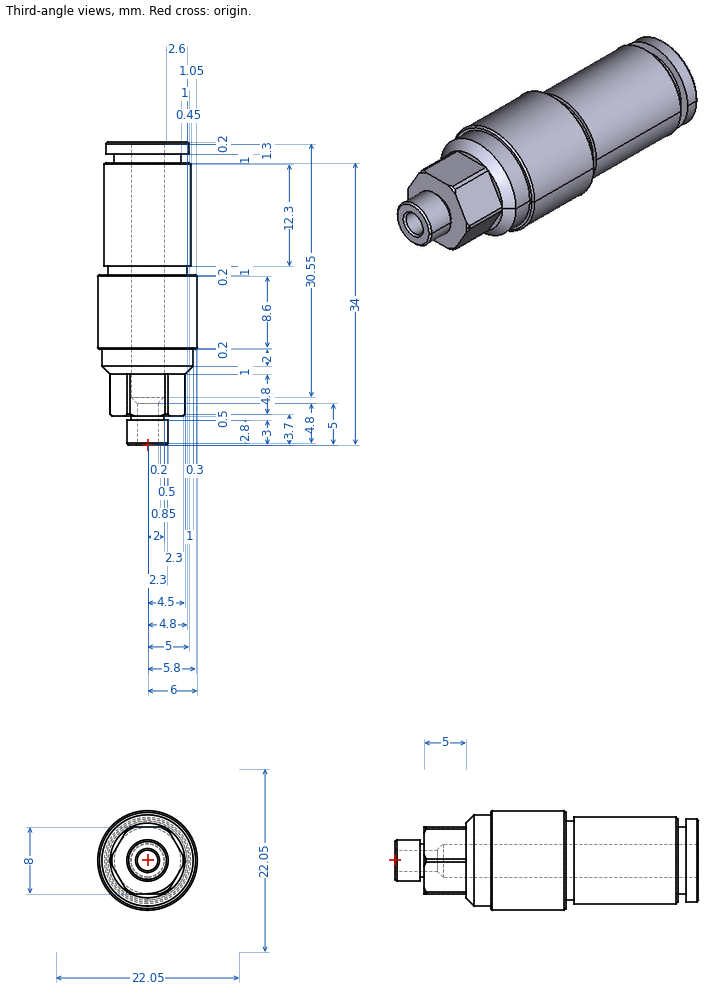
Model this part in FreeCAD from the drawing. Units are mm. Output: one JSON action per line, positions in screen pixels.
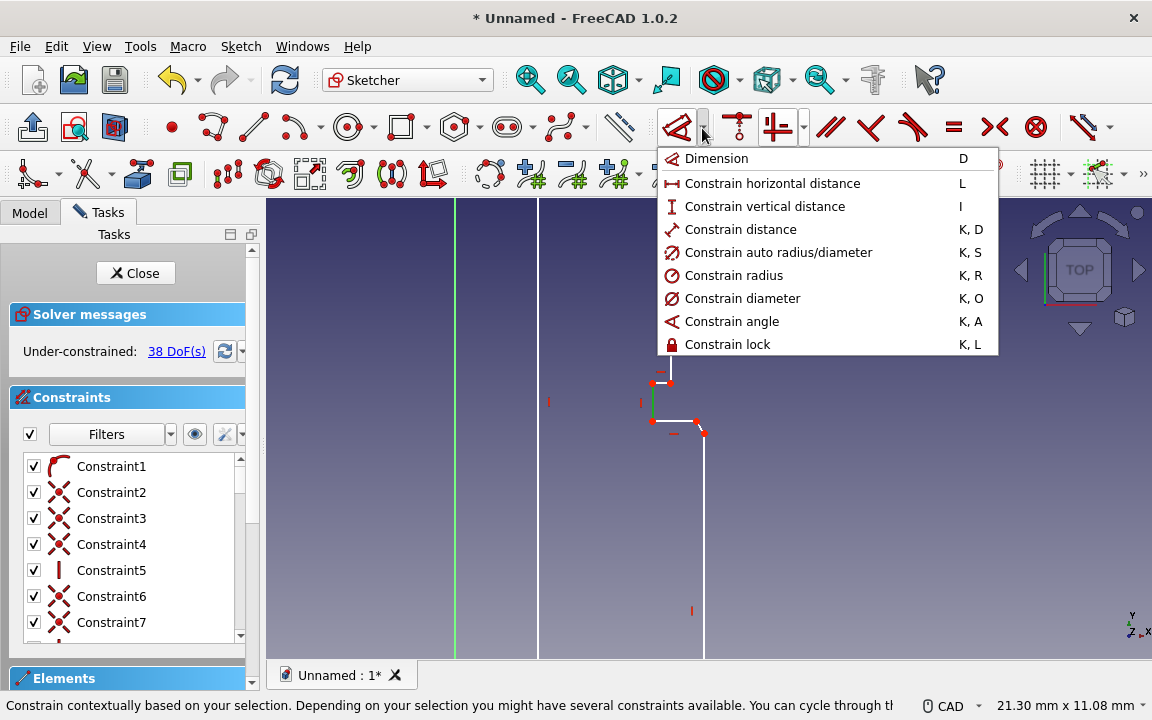
{"action": "left_click", "coordinate": [828, 206]}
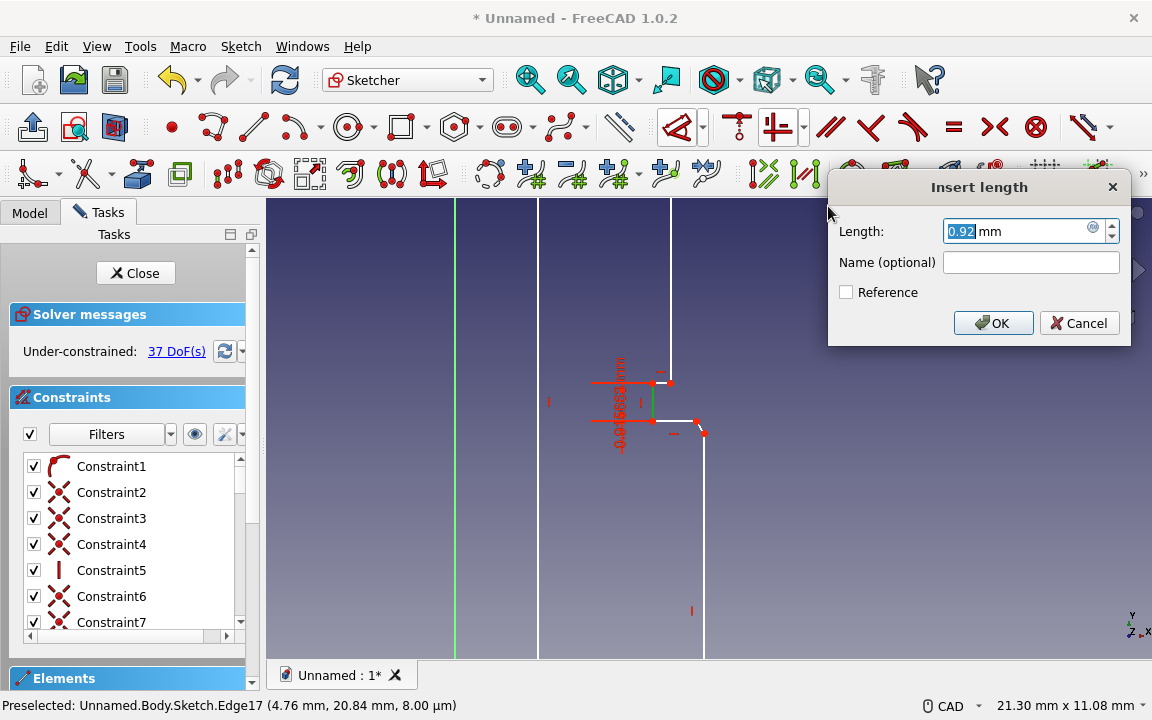
{"action": "type", "text": "1"}
{"action": "key", "text": "Return"}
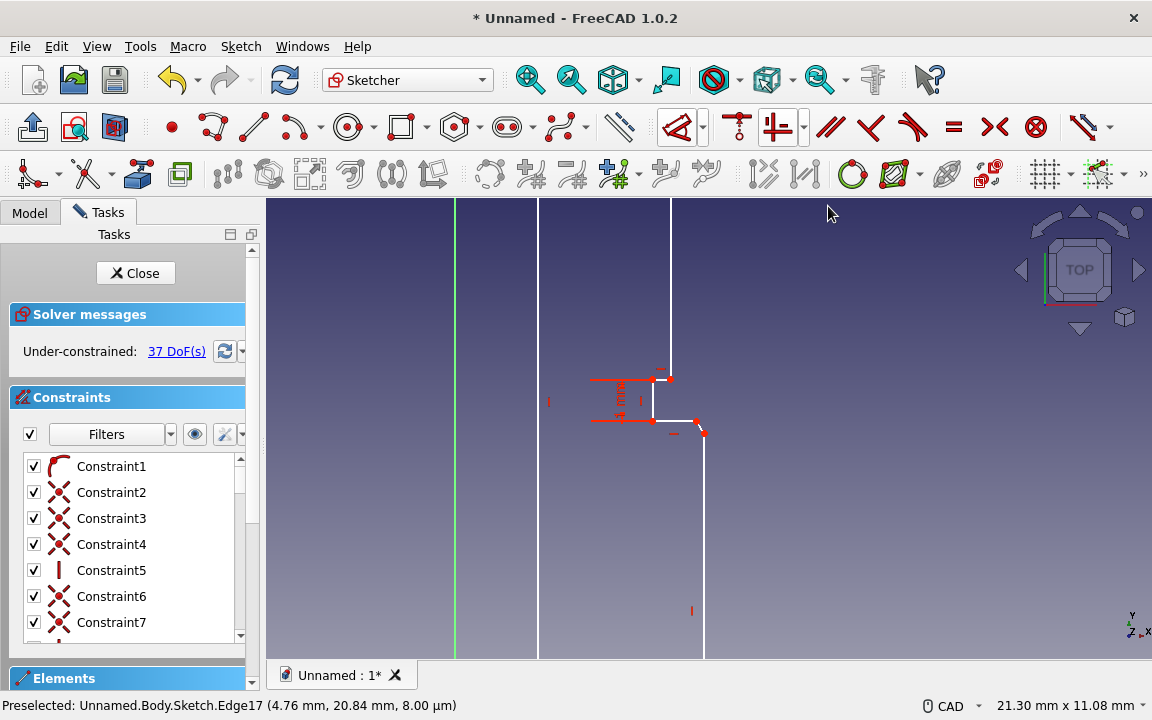
{"action": "scroll", "coordinate": [656, 407], "scroll_direction": "down", "scroll_amount": 8}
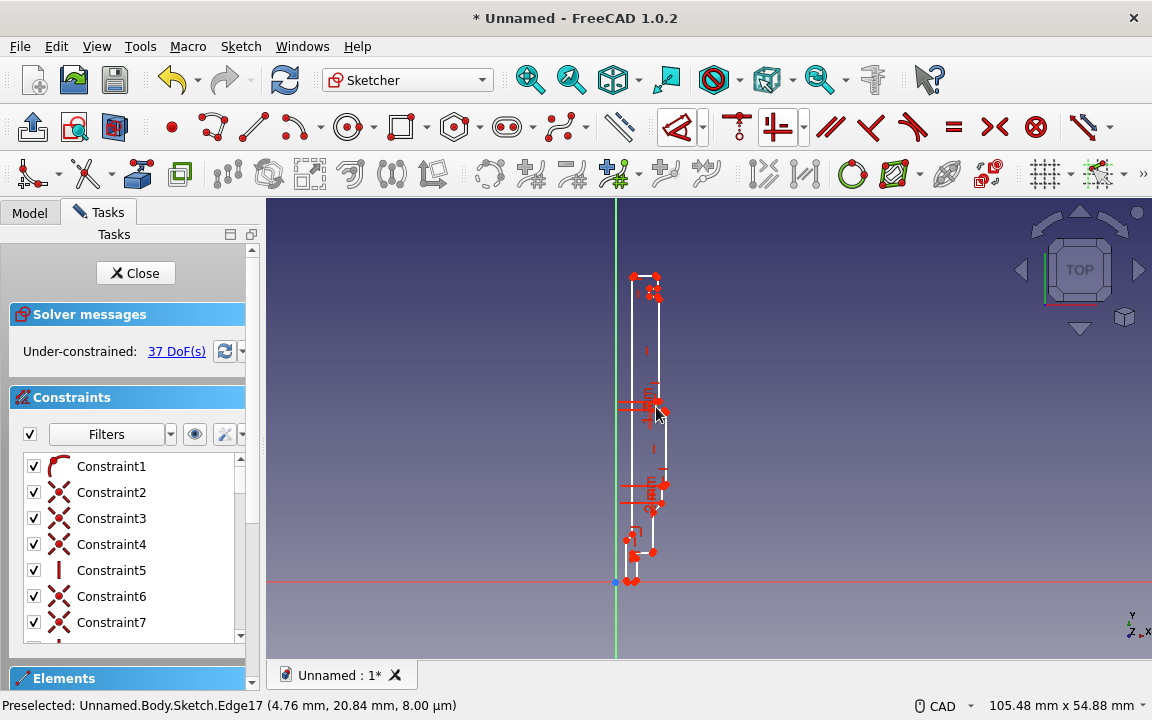
{"action": "scroll", "coordinate": [655, 297], "scroll_direction": "up", "scroll_amount": 9}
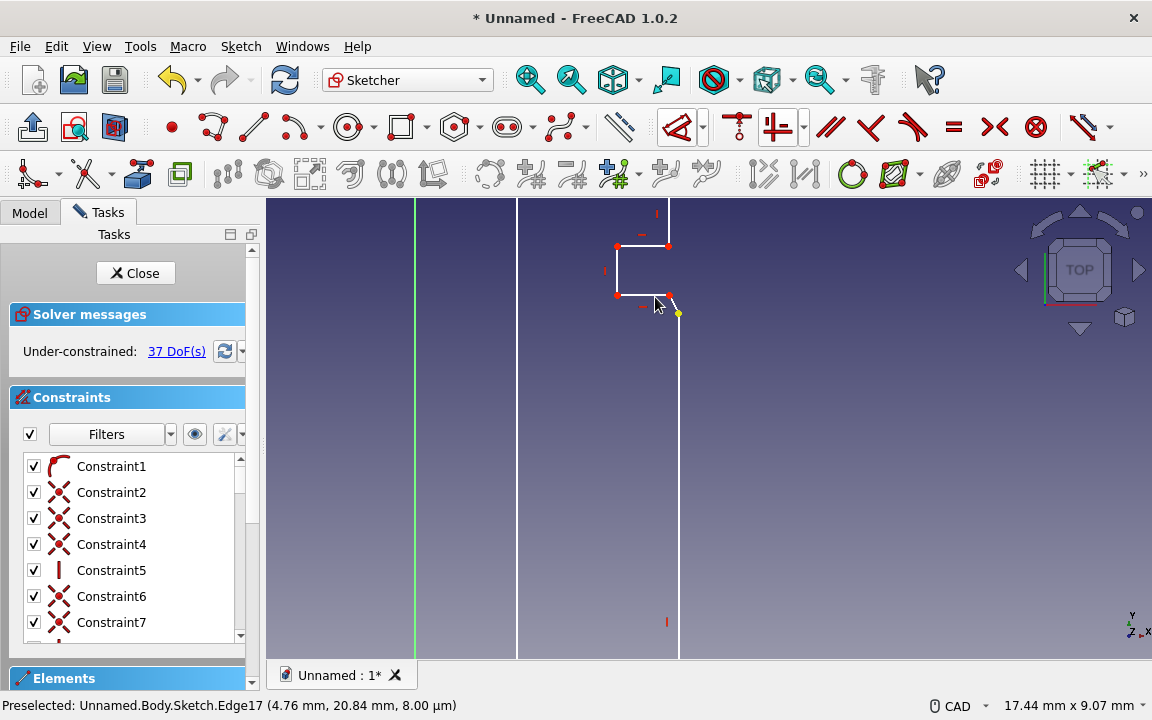
{"action": "left_click", "coordinate": [654, 295]}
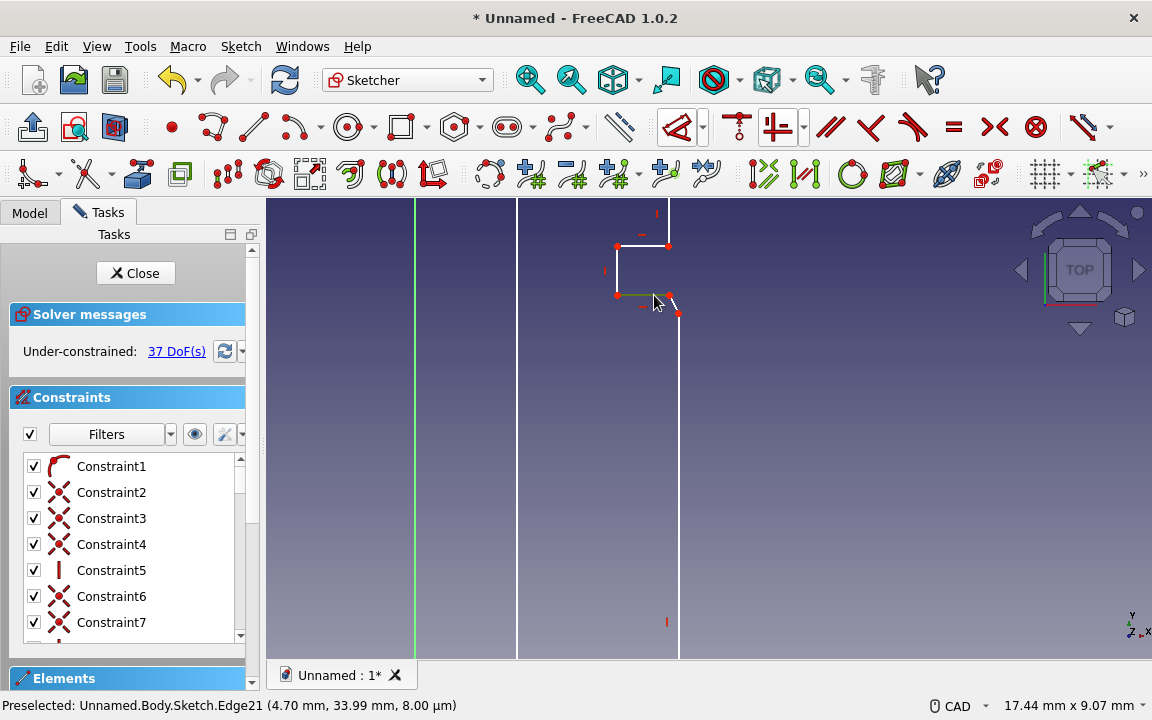
{"action": "key", "text": "l"}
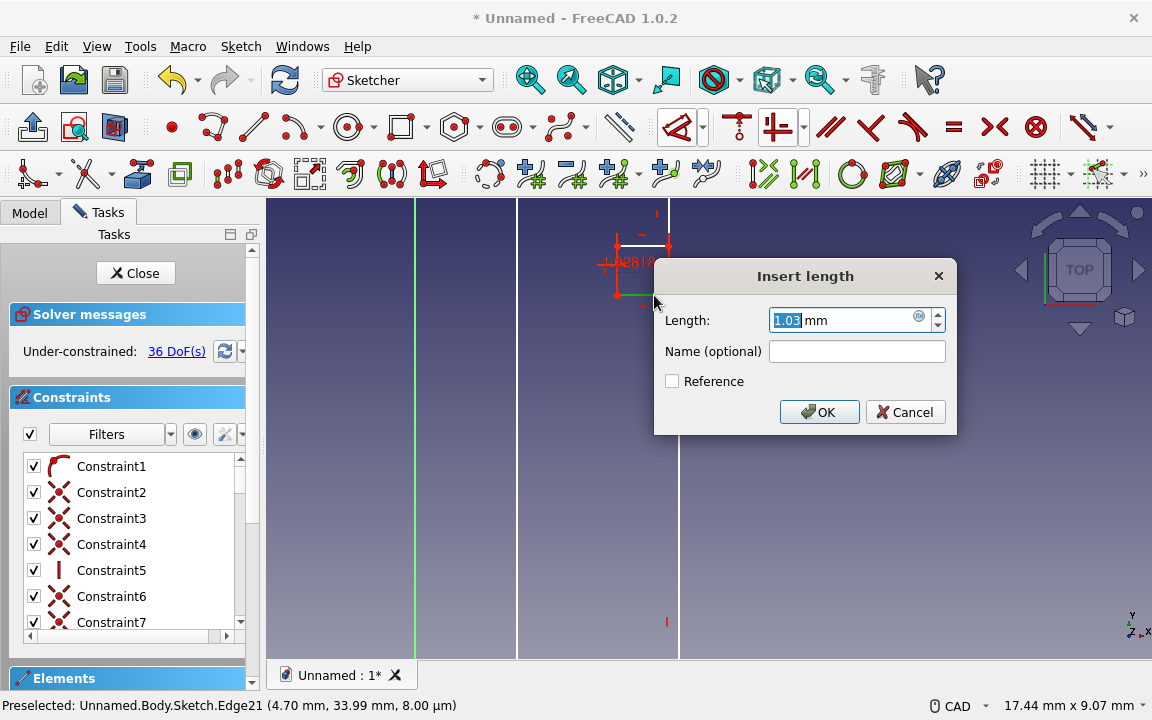
{"action": "type", "text": "1"}
{"action": "key", "text": "Return"}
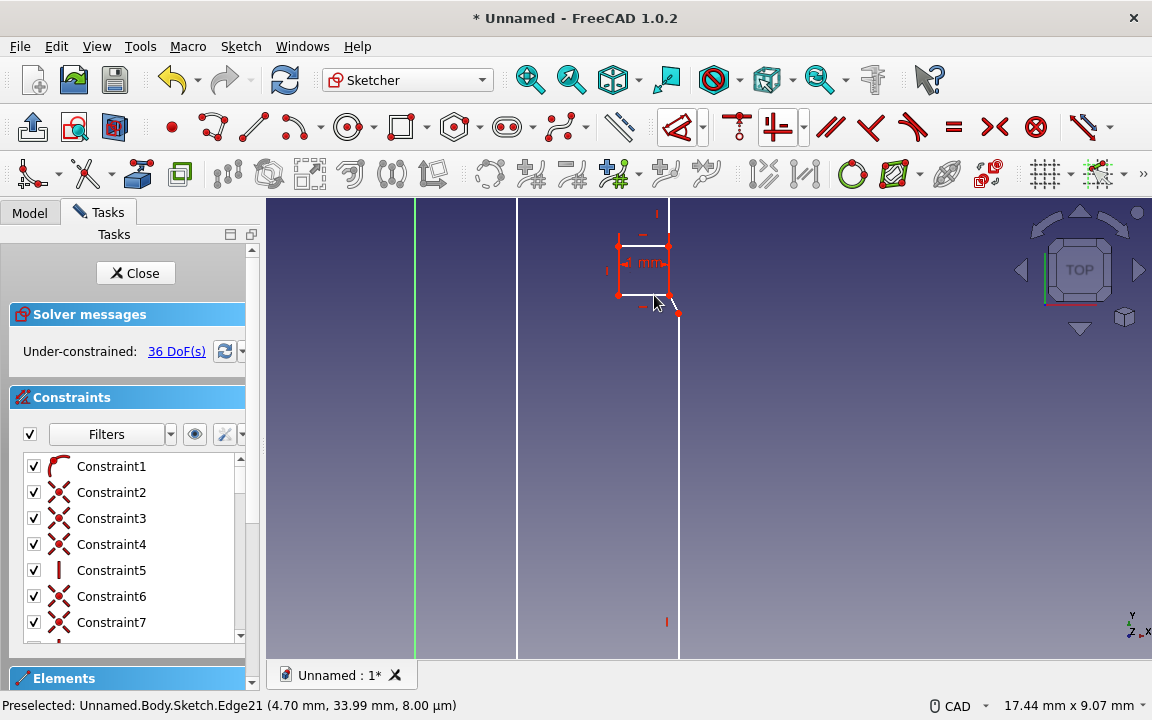
{"action": "left_click", "coordinate": [619, 281]}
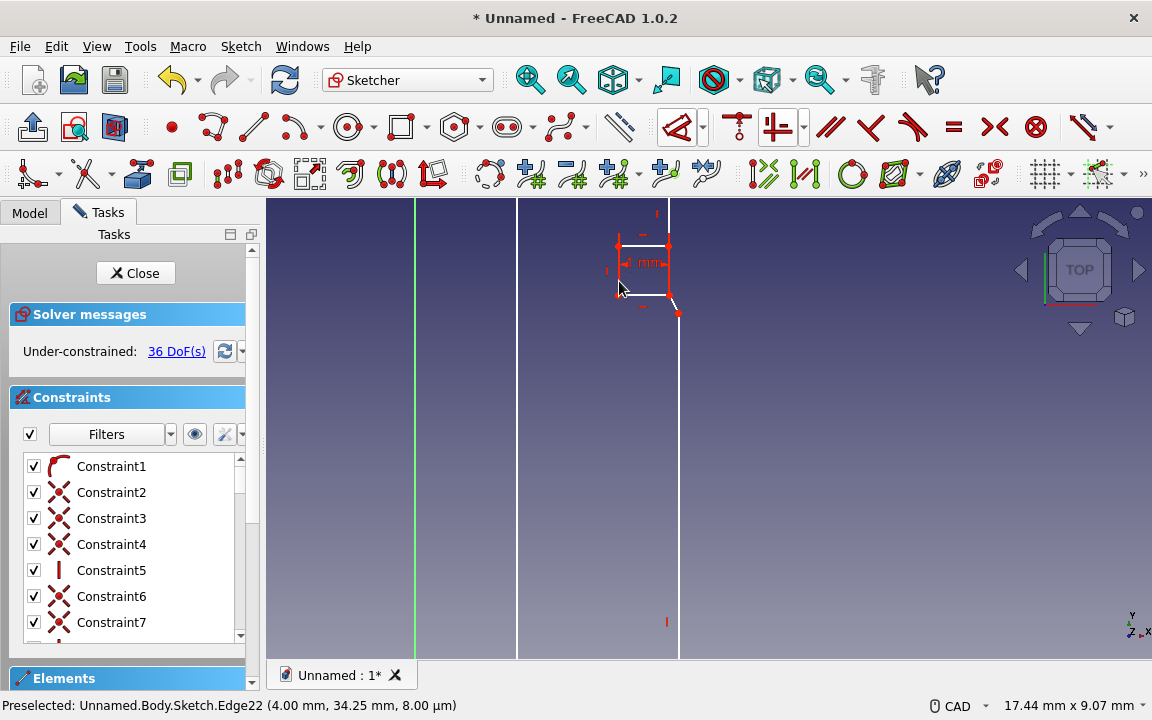
{"action": "left_click", "coordinate": [702, 128]}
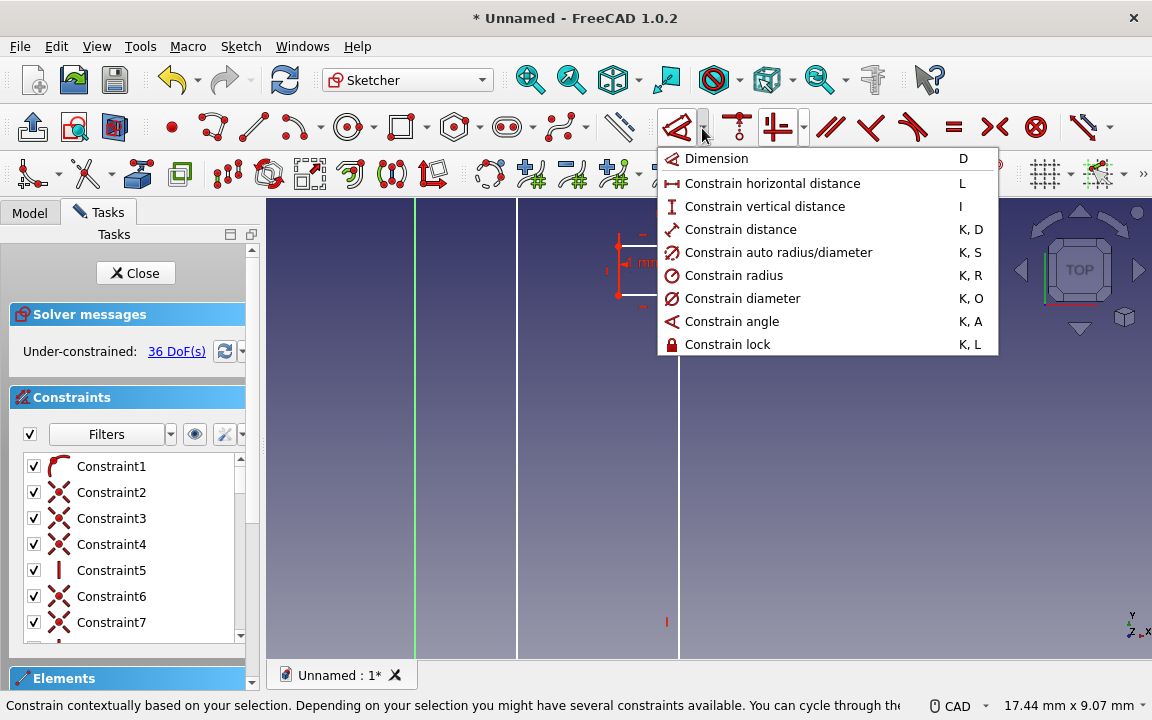
{"action": "left_click", "coordinate": [828, 206]}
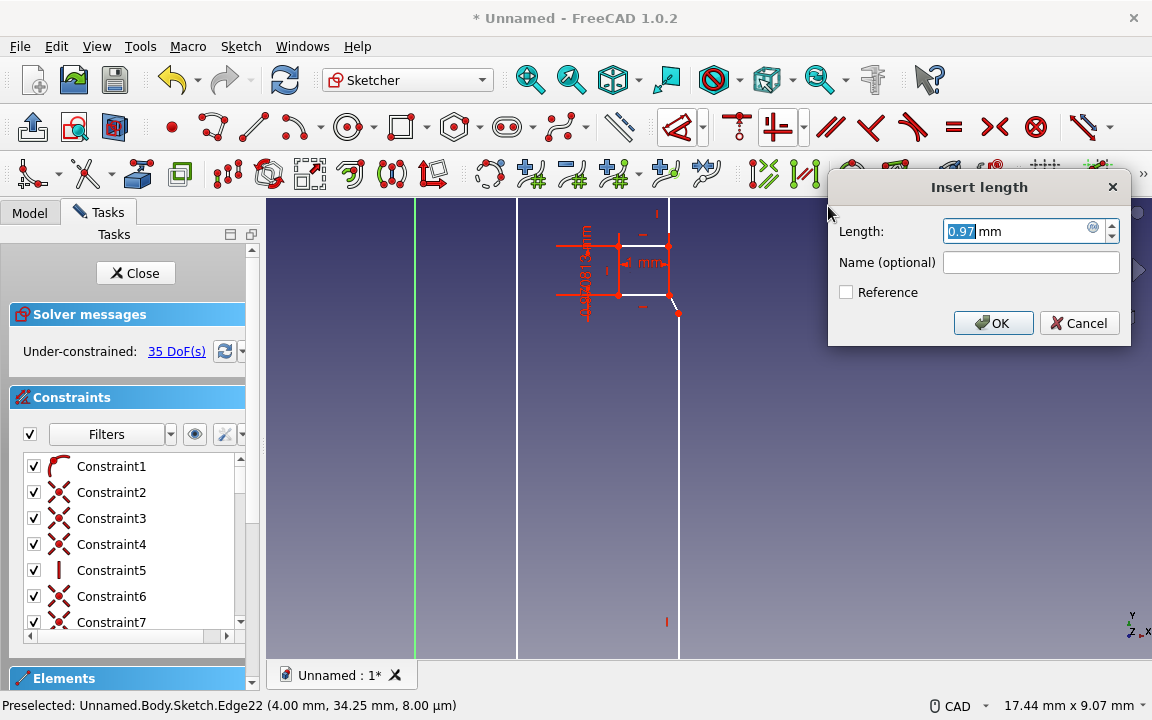
{"action": "type", "text": "1"}
{"action": "key", "text": "Return"}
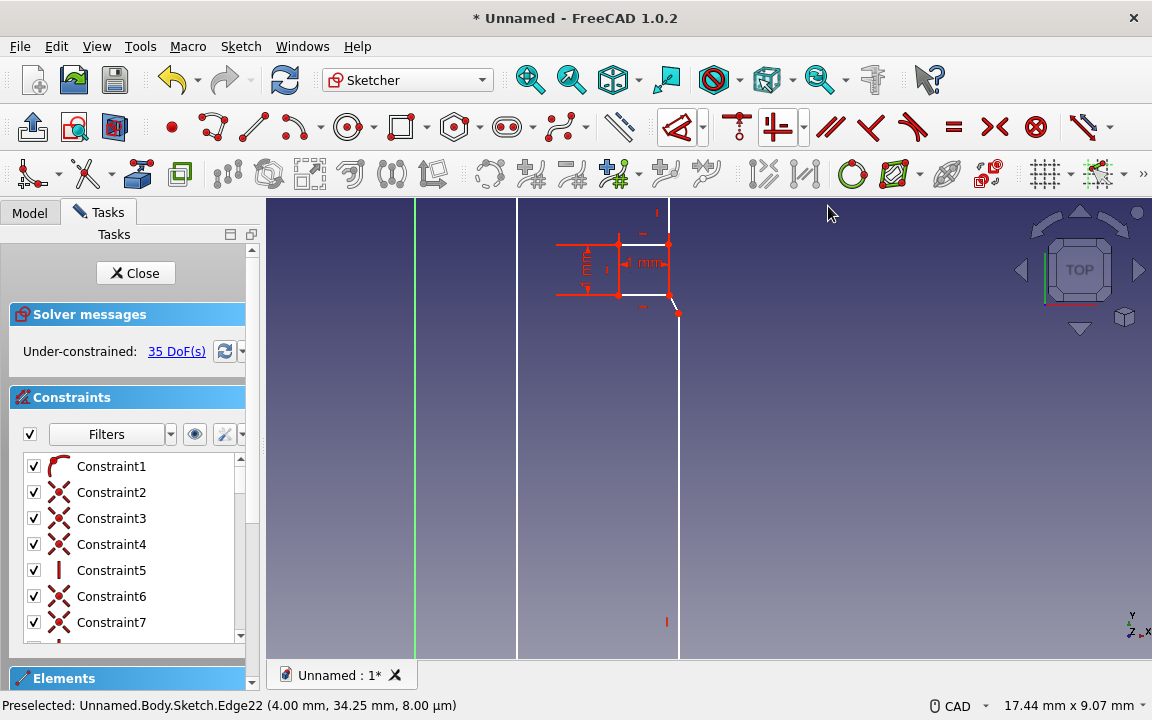
{"action": "left_click", "coordinate": [634, 245]}